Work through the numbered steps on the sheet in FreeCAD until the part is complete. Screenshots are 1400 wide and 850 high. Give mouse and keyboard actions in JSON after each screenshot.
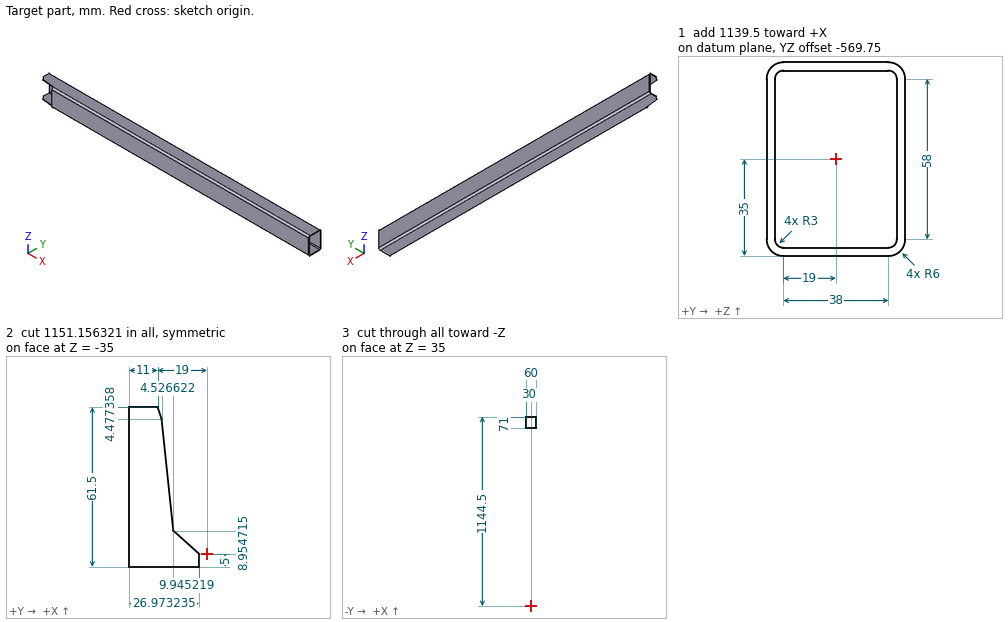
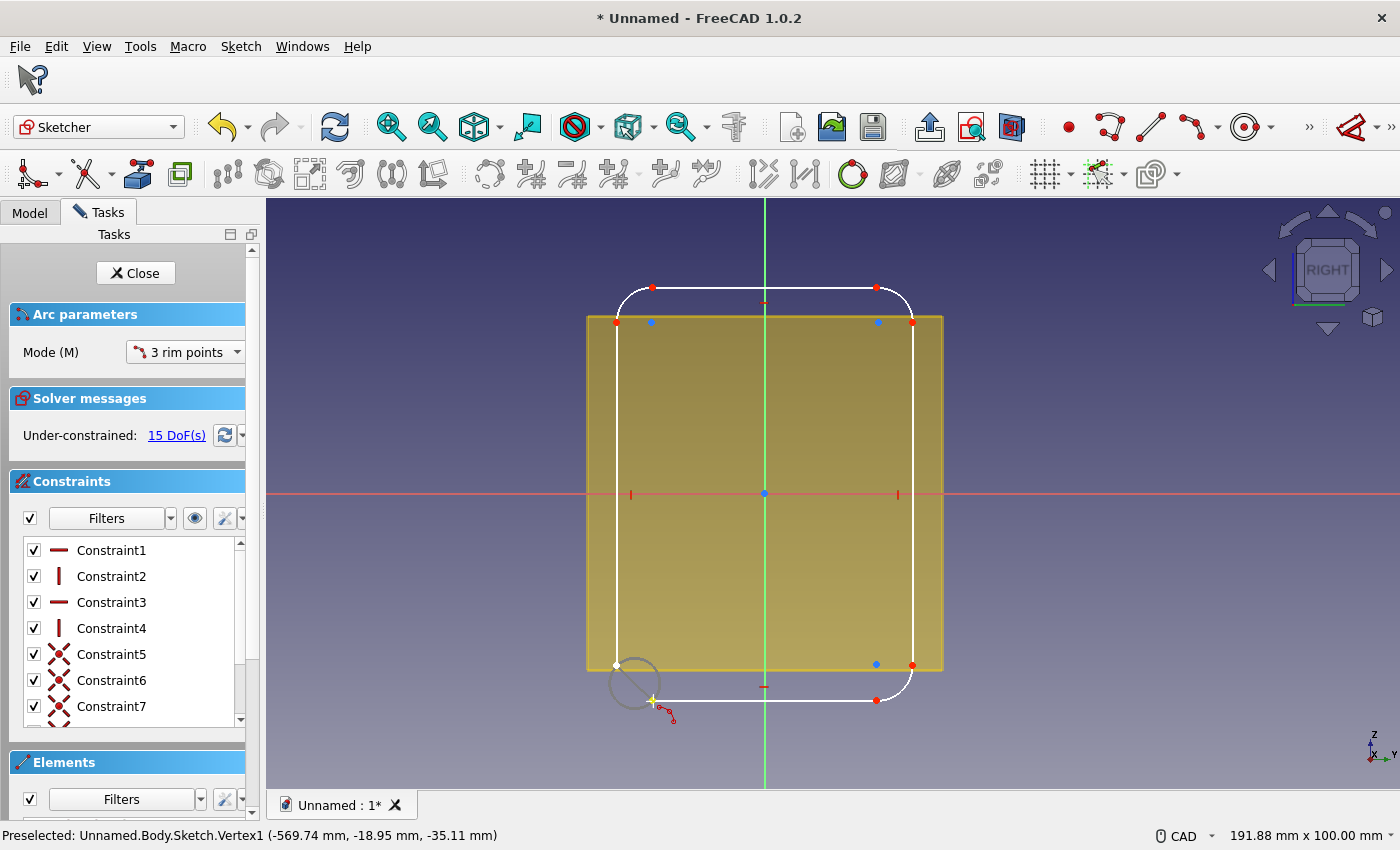
{"action": "scroll", "coordinate": [627, 690], "scroll_direction": "up", "scroll_amount": 3}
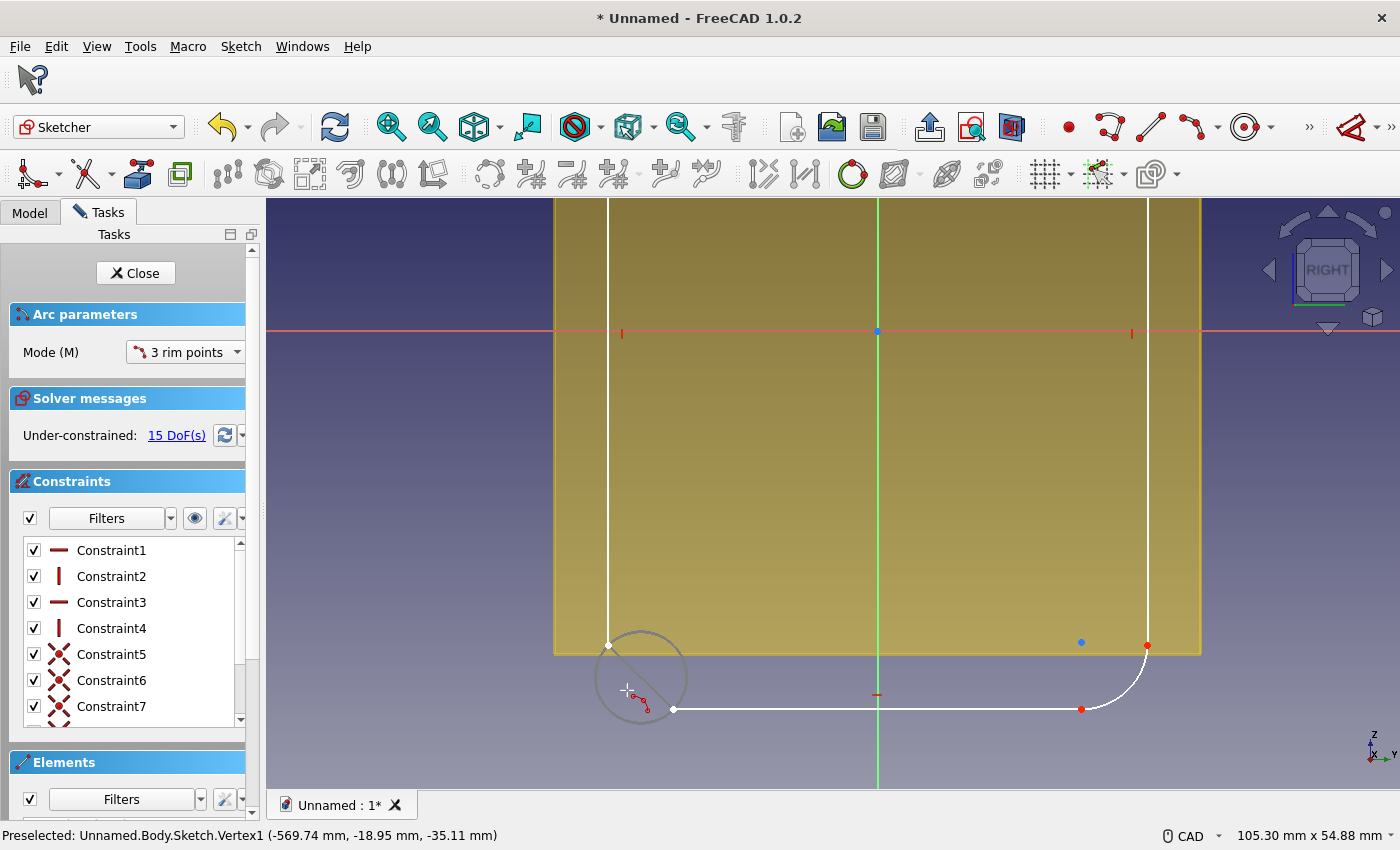
{"action": "left_click", "coordinate": [628, 689]}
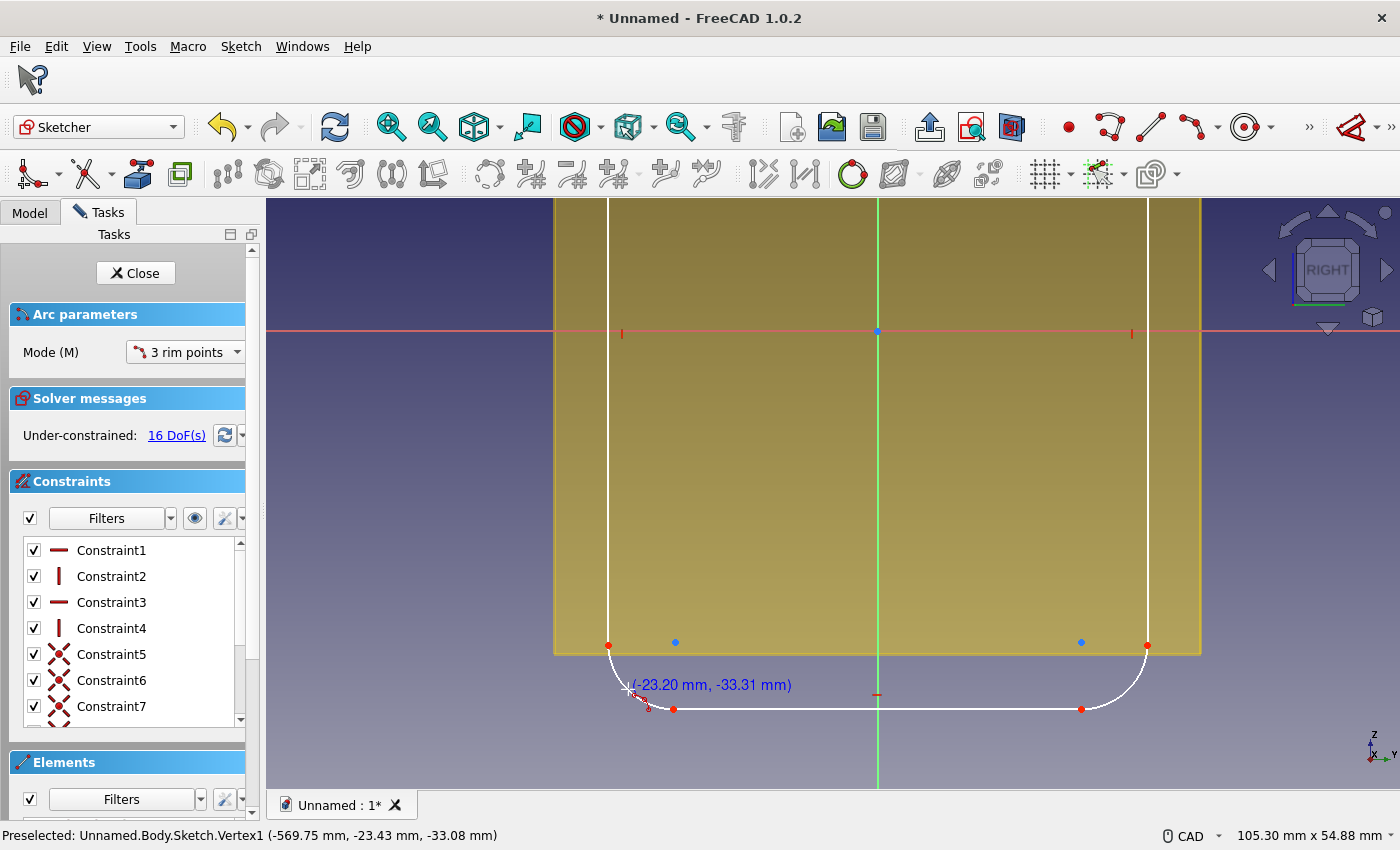
{"action": "key", "text": "g l"}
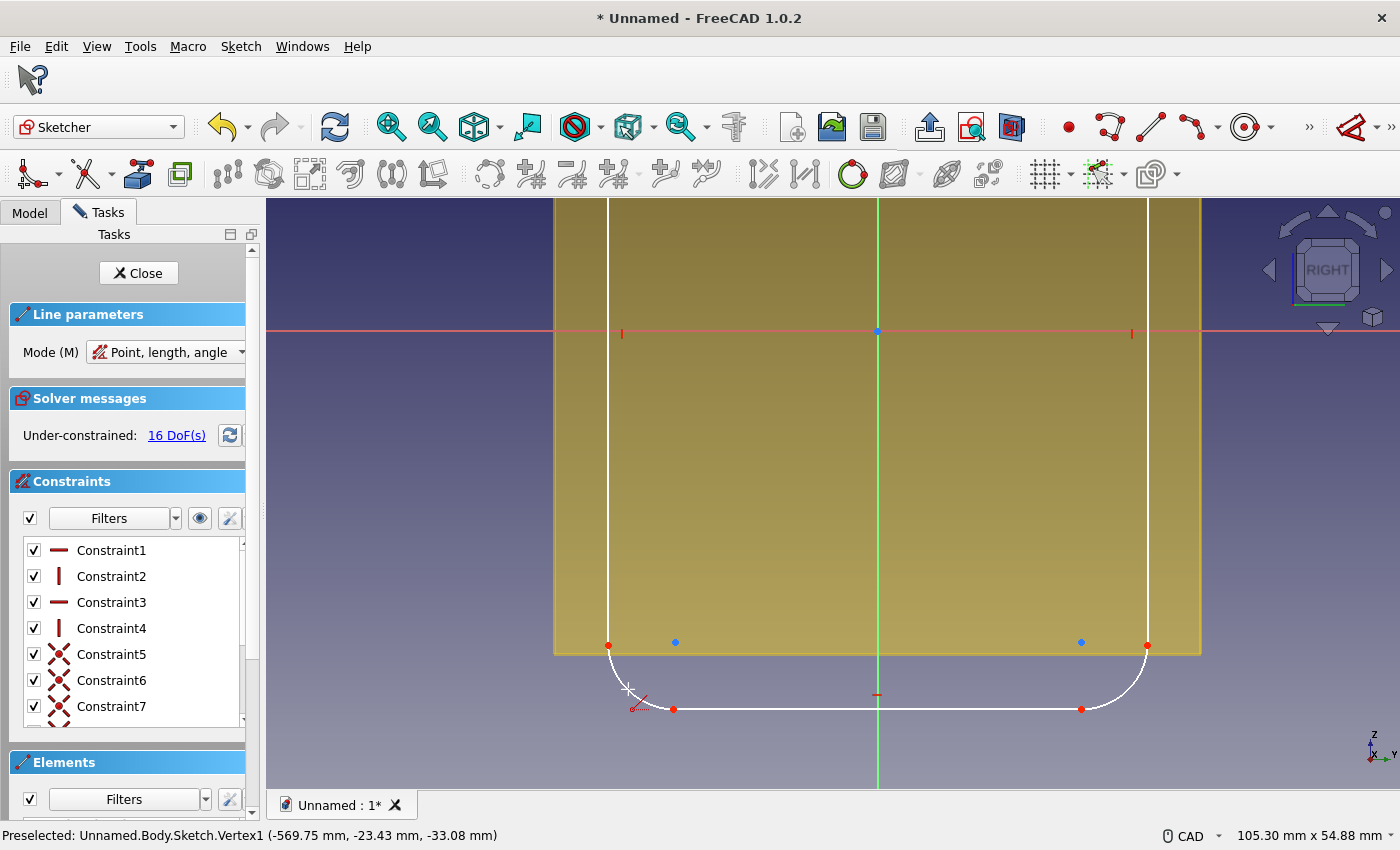
{"action": "left_click", "coordinate": [1082, 676]}
{"action": "left_click", "coordinate": [673, 676]}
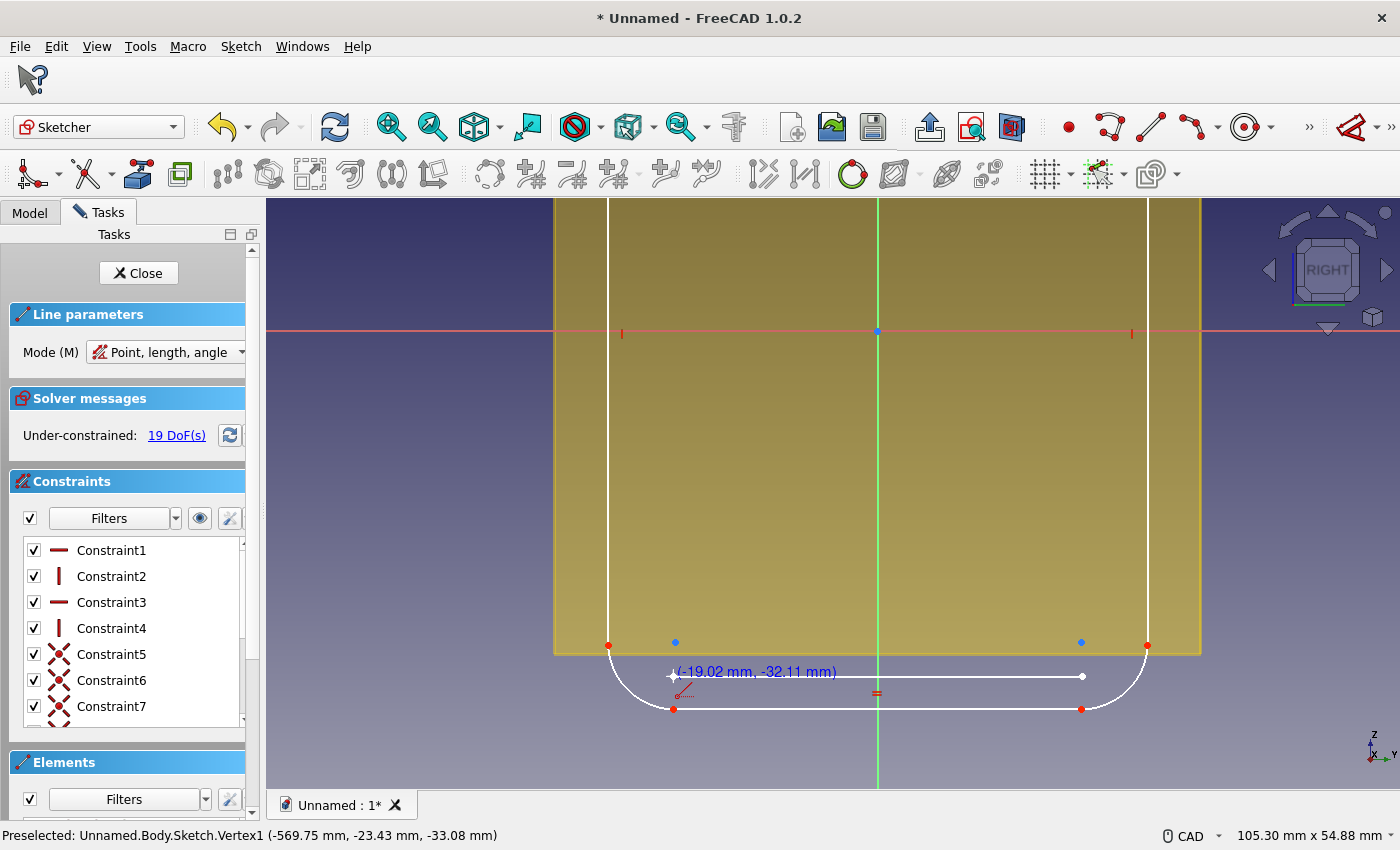
{"action": "left_click", "coordinate": [641, 644]}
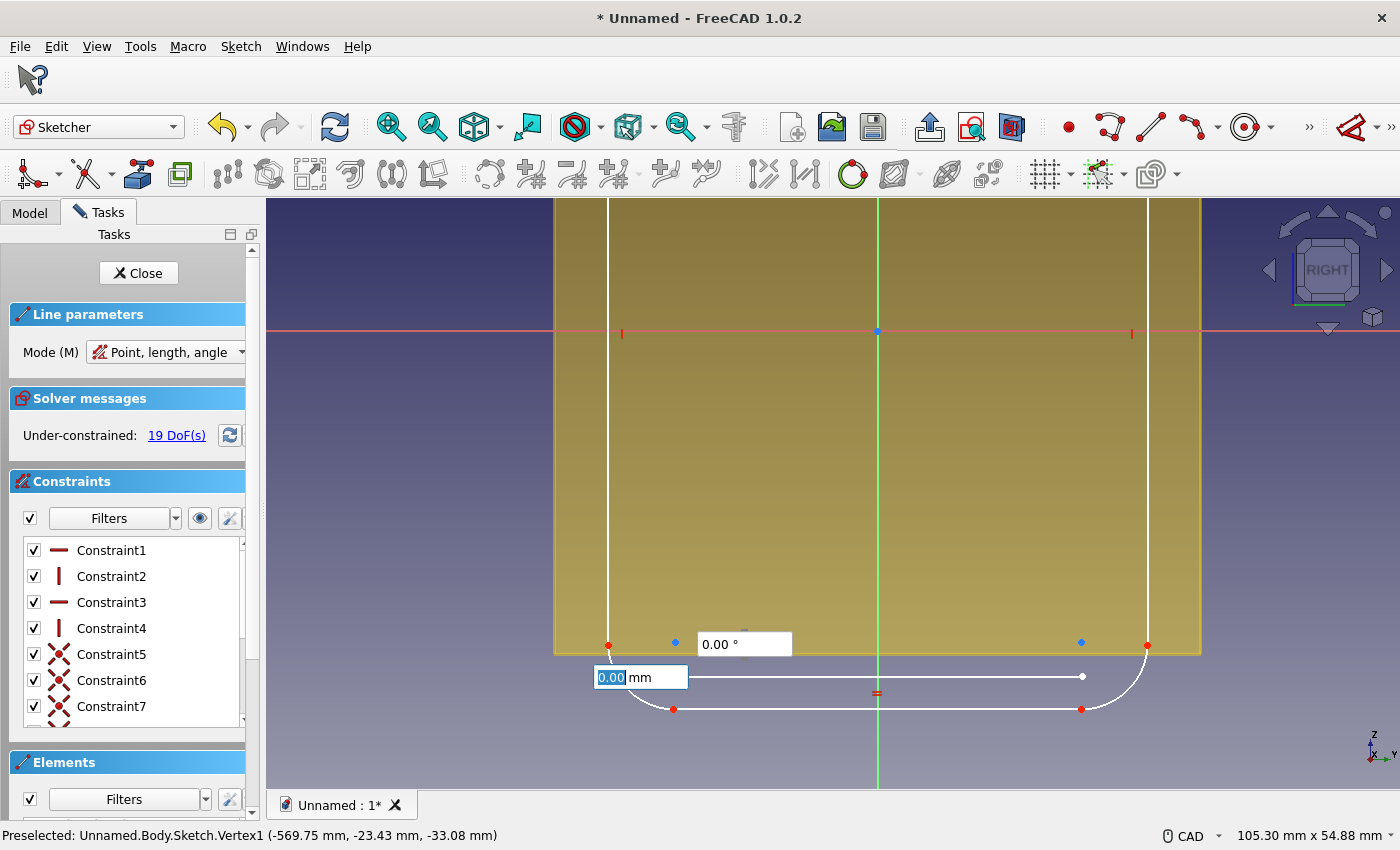
{"action": "scroll", "coordinate": [627, 691], "scroll_direction": "down", "scroll_amount": 3}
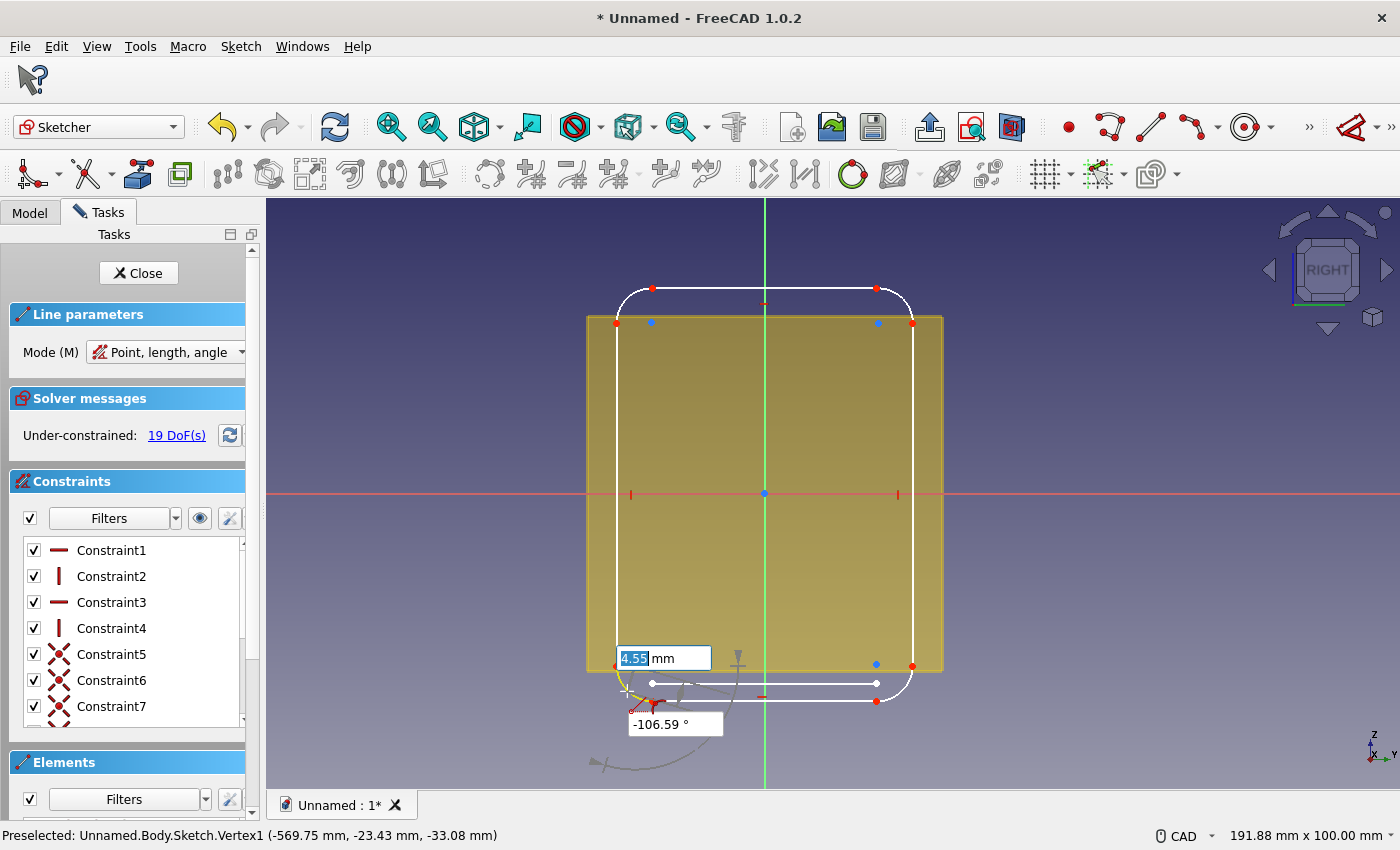
{"action": "left_click", "coordinate": [635, 323]}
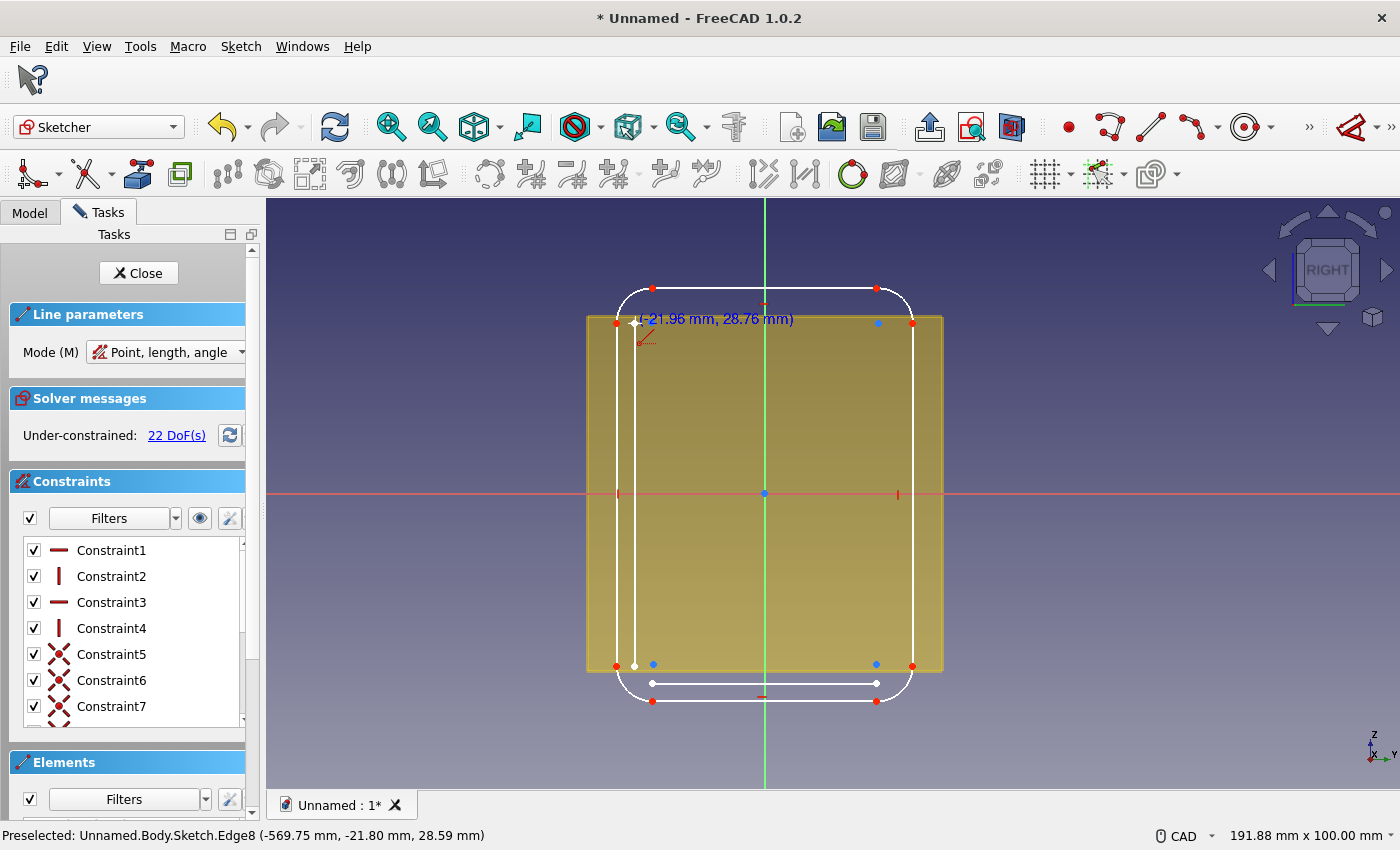
{"action": "left_click", "coordinate": [653, 305]}
{"action": "left_click", "coordinate": [877, 305]}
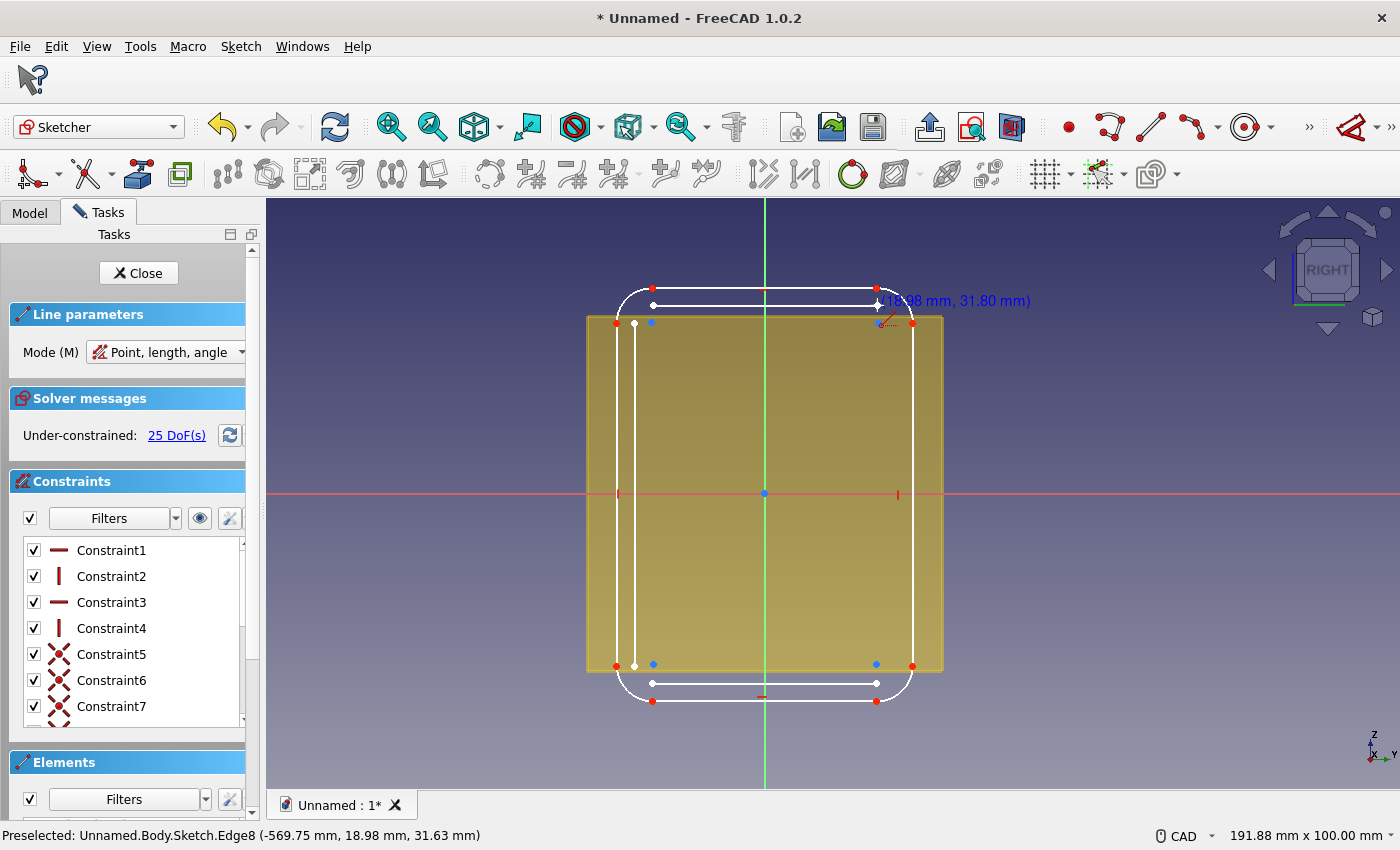
{"action": "left_click", "coordinate": [895, 323]}
{"action": "left_click", "coordinate": [895, 665]}